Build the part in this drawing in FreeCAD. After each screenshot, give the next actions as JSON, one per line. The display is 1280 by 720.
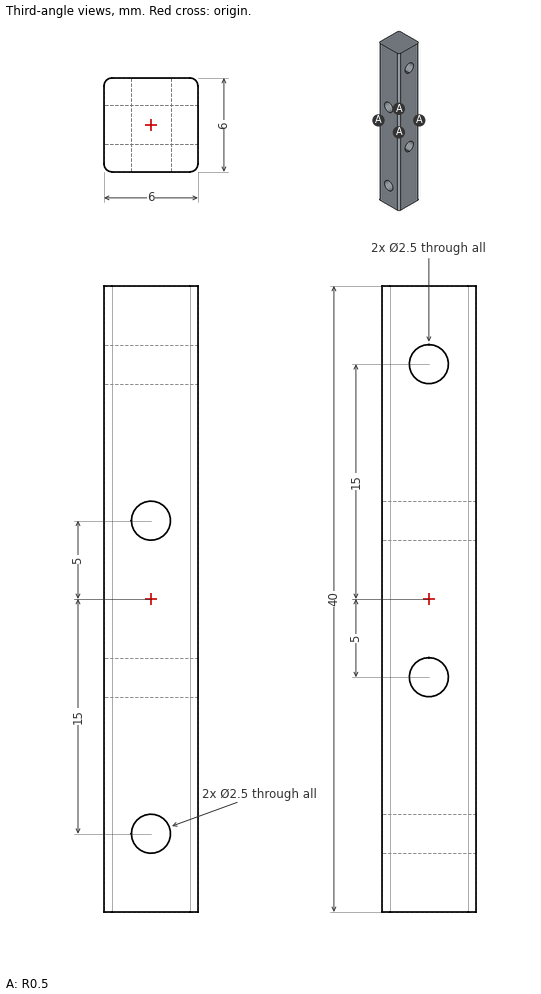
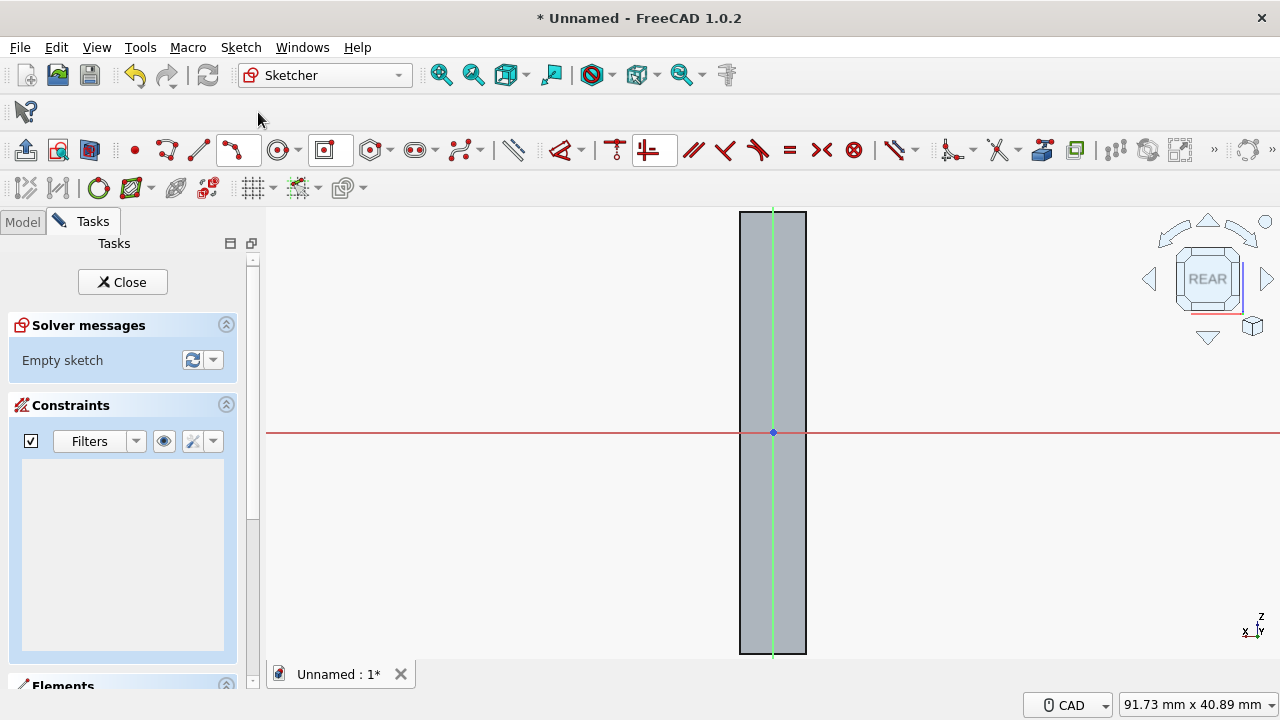
{"action": "scroll", "coordinate": [395, 235], "scroll_direction": "down", "scroll_amount": 1}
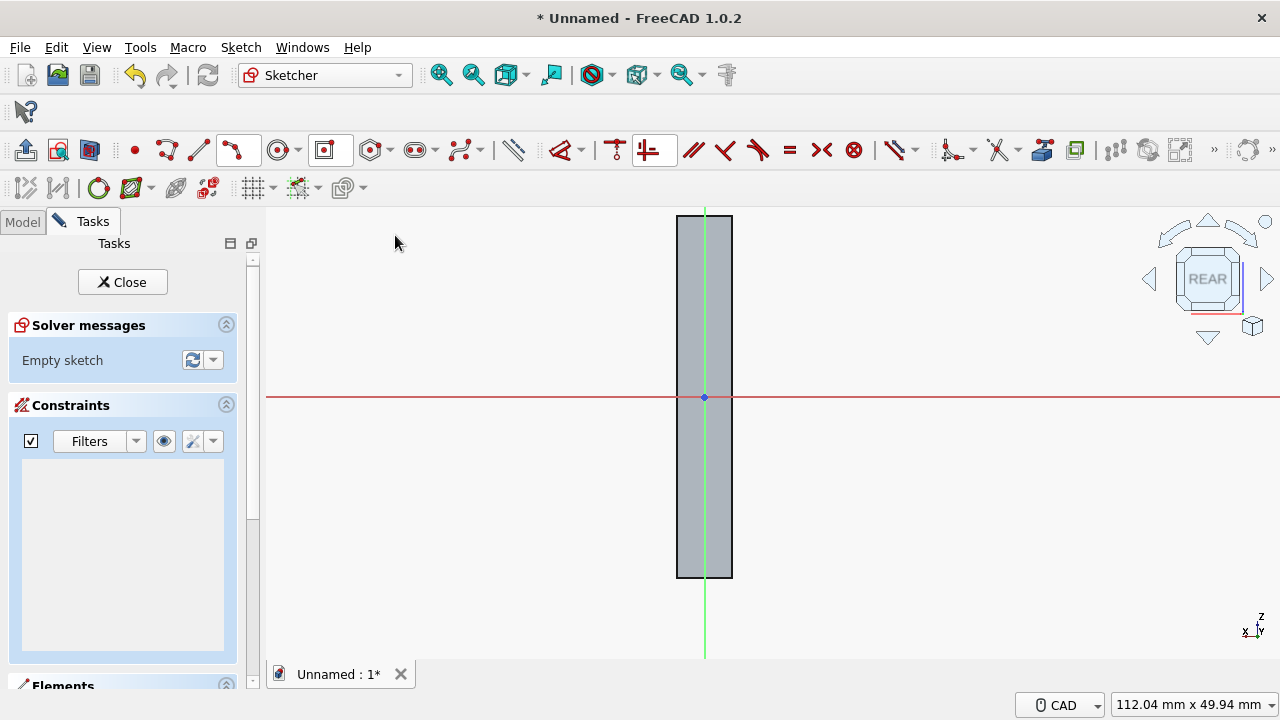
{"action": "scroll", "coordinate": [705, 461], "scroll_direction": "up", "scroll_amount": 2}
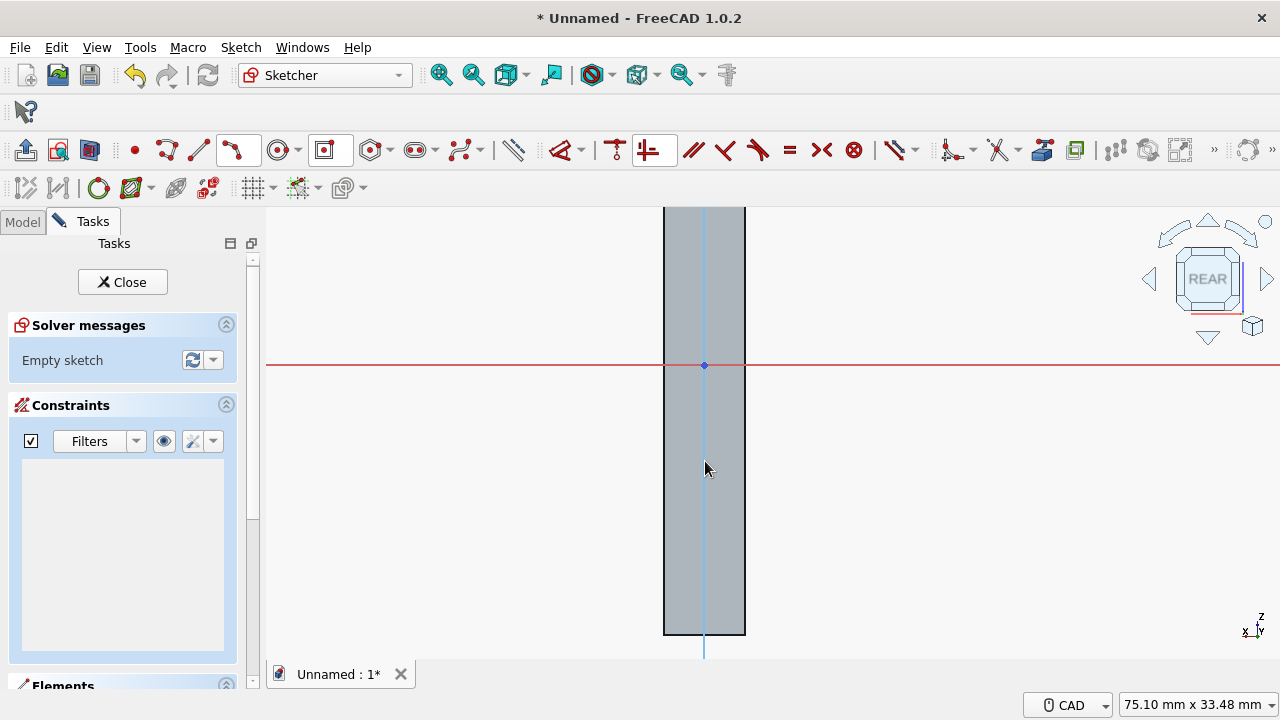
{"action": "left_click", "coordinate": [278, 150]}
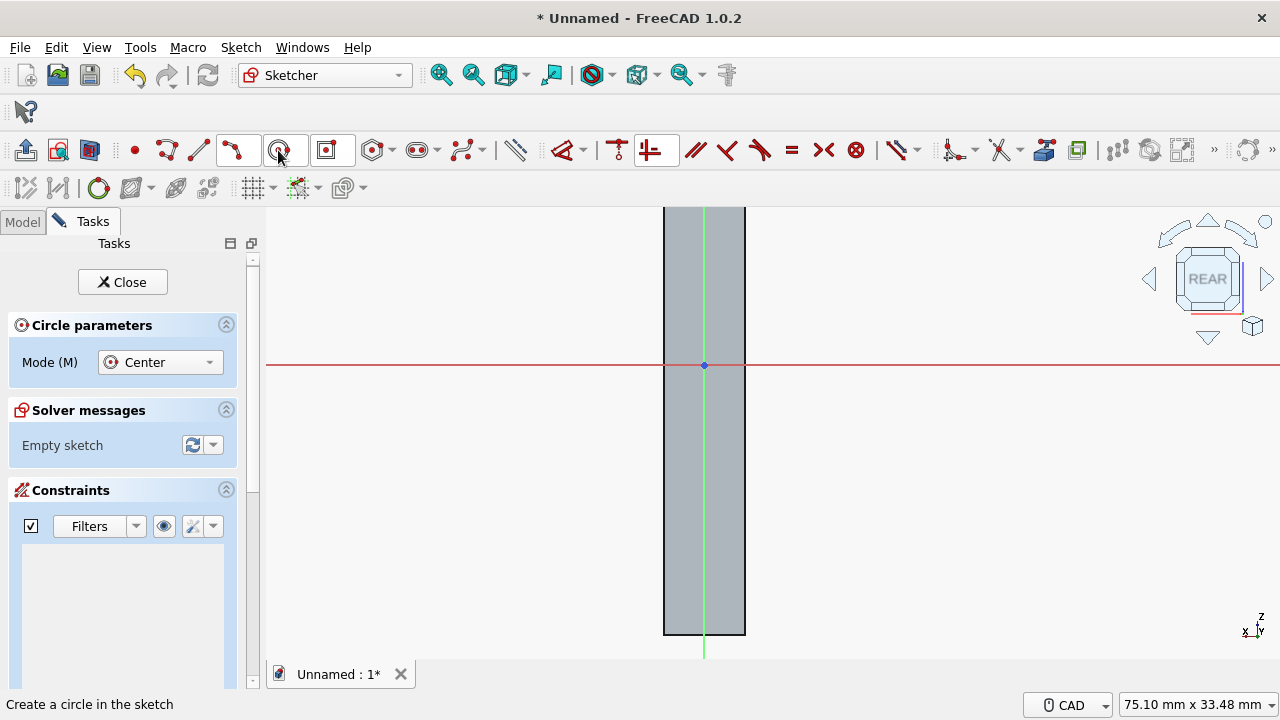
{"action": "scroll", "coordinate": [704, 568], "scroll_direction": "up", "scroll_amount": 2}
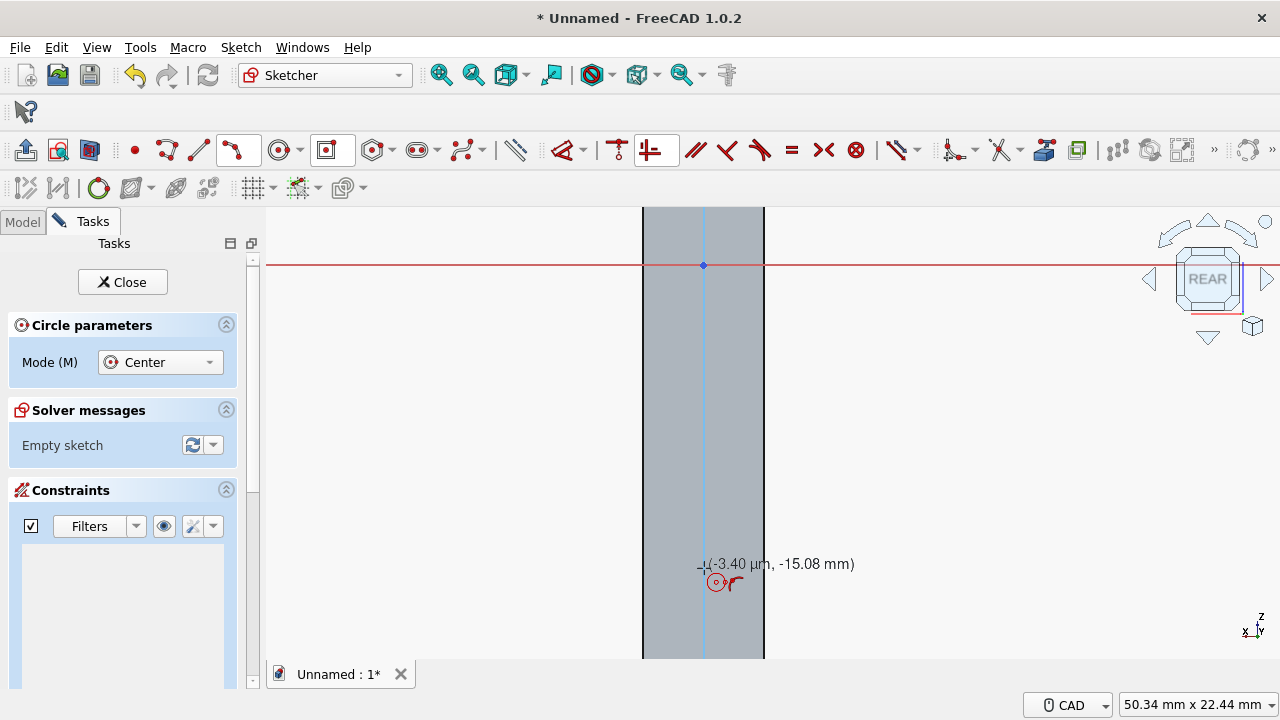
{"action": "left_click", "coordinate": [704, 568]}
{"action": "left_click", "coordinate": [722, 550]}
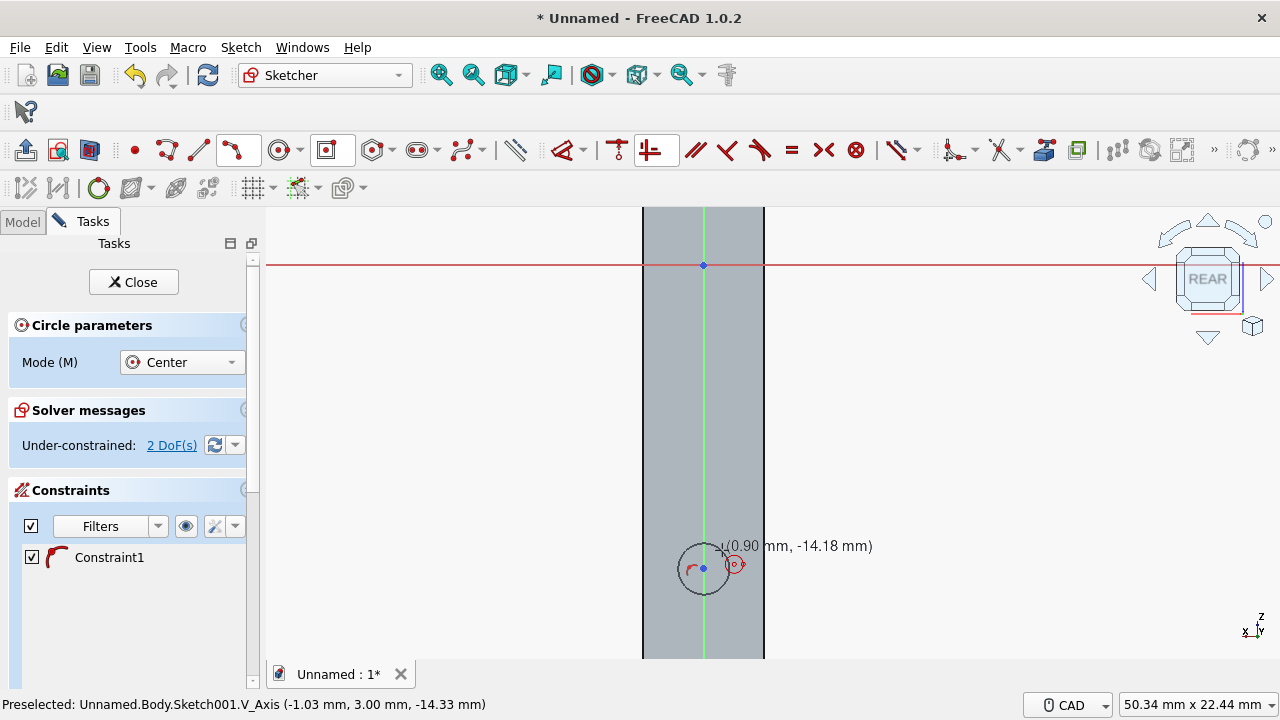
{"action": "scroll", "coordinate": [706, 569], "scroll_direction": "down", "scroll_amount": 2}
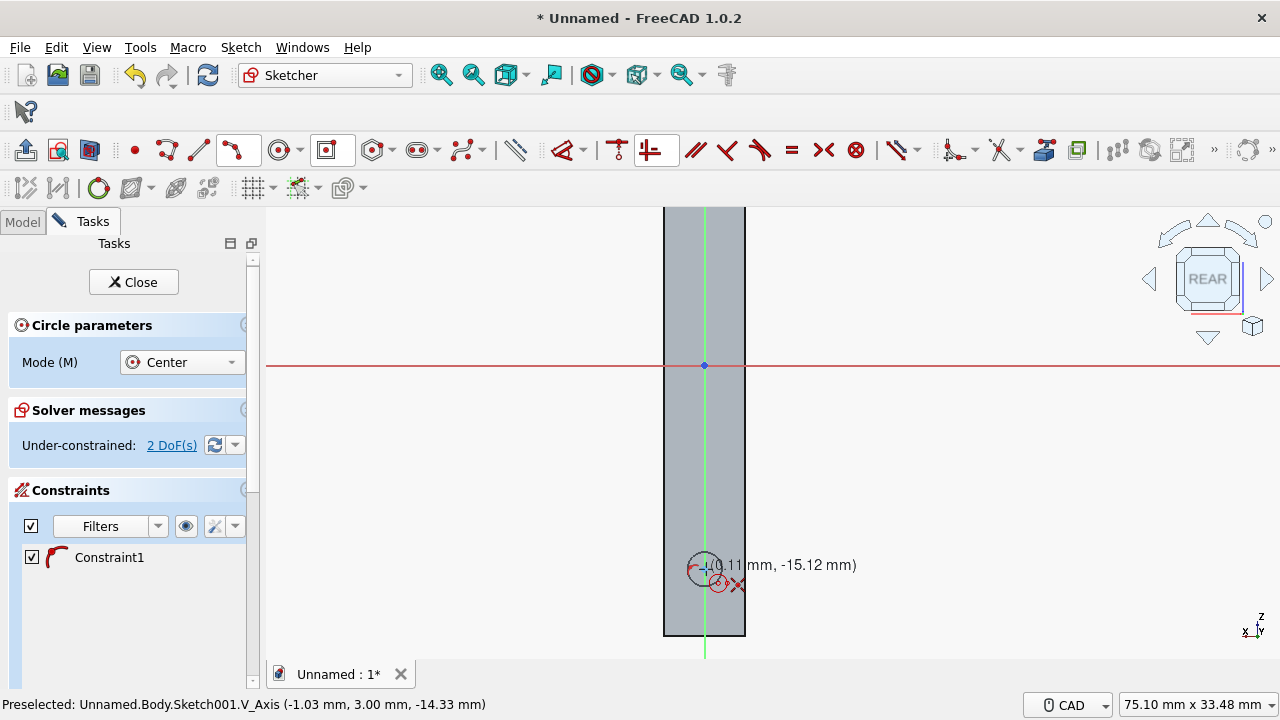
{"action": "scroll", "coordinate": [705, 298], "scroll_direction": "up", "scroll_amount": 2}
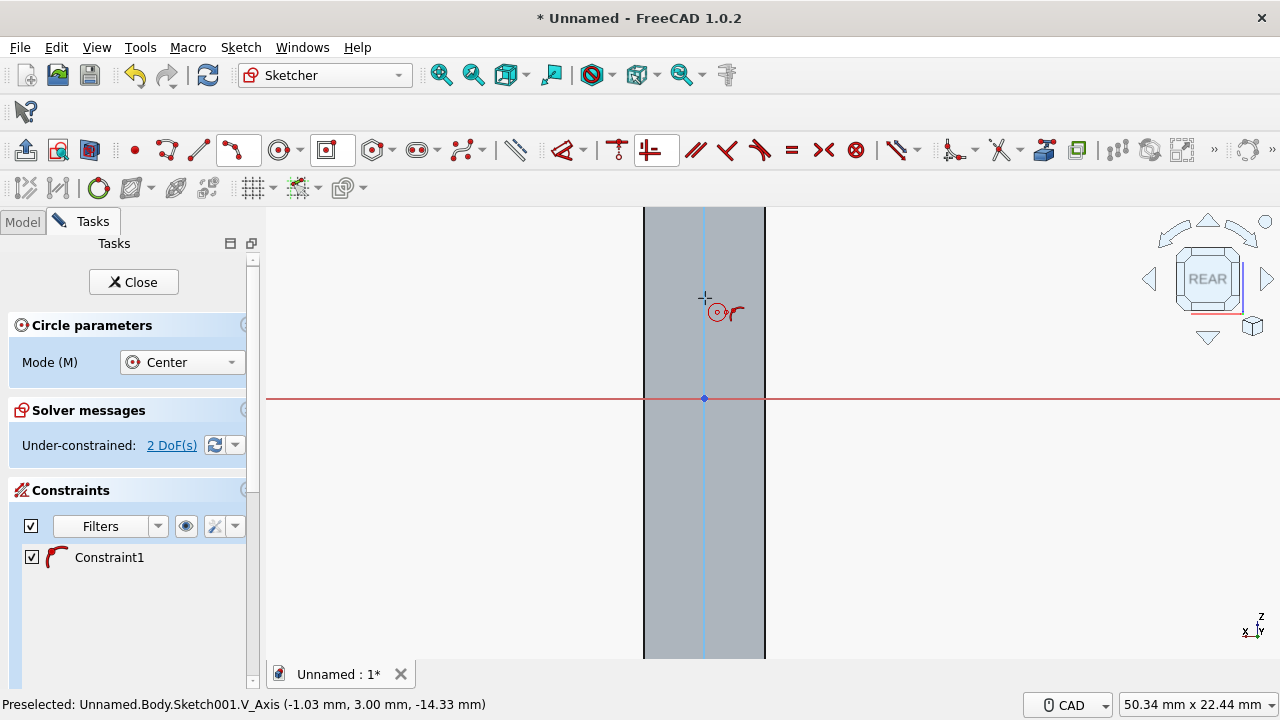
{"action": "left_click", "coordinate": [704, 298]}
{"action": "left_click", "coordinate": [722, 280]}
{"action": "key", "text": "Escape"}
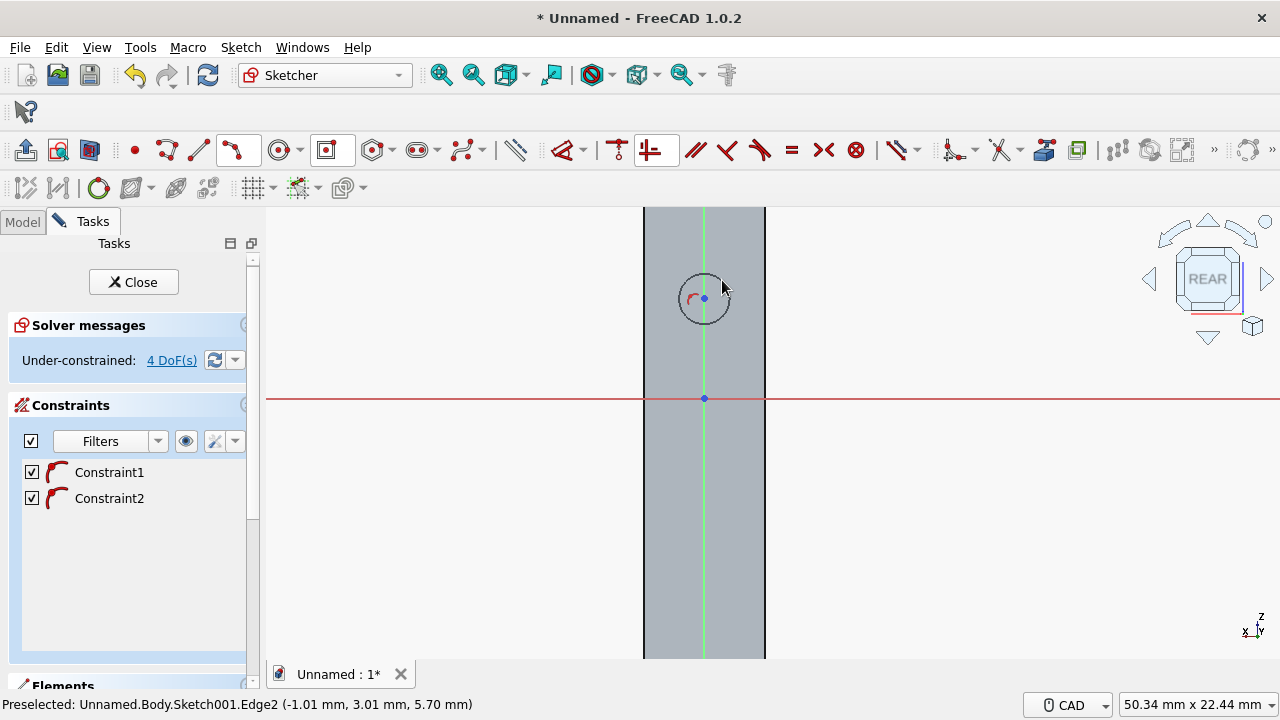
{"action": "scroll", "coordinate": [705, 297], "scroll_direction": "down", "scroll_amount": 2}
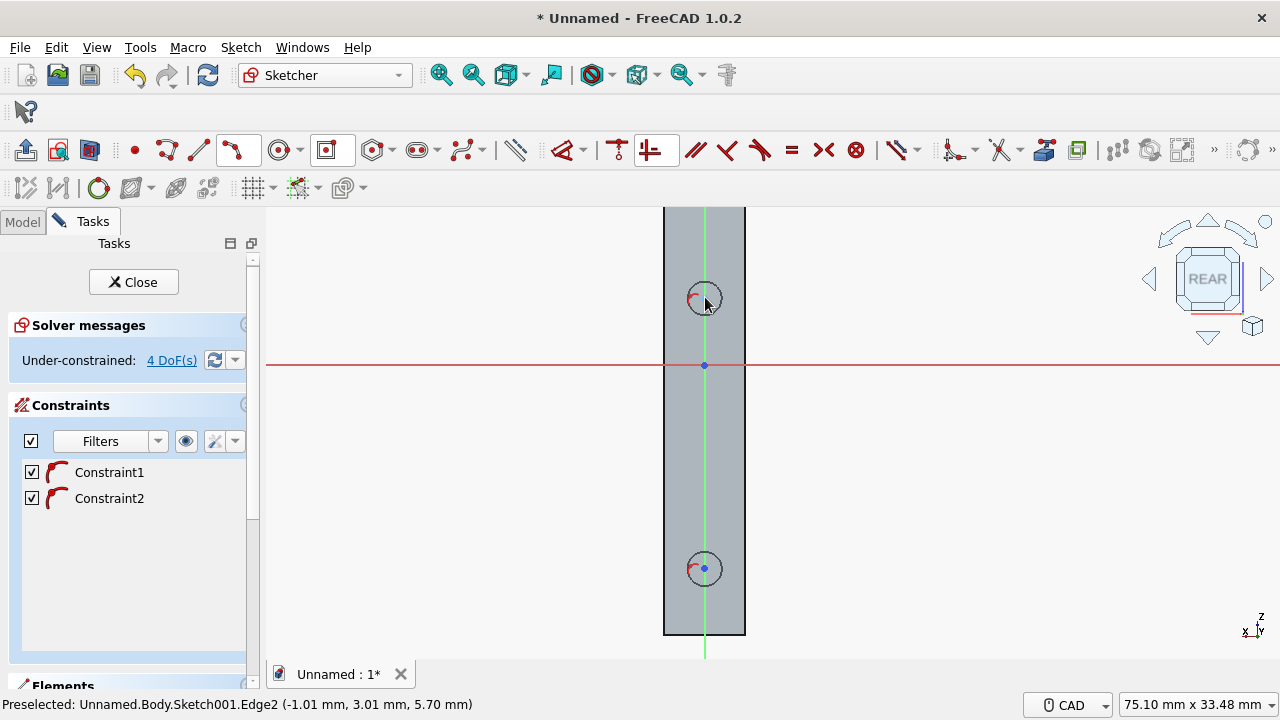
{"action": "left_click", "coordinate": [717, 557]}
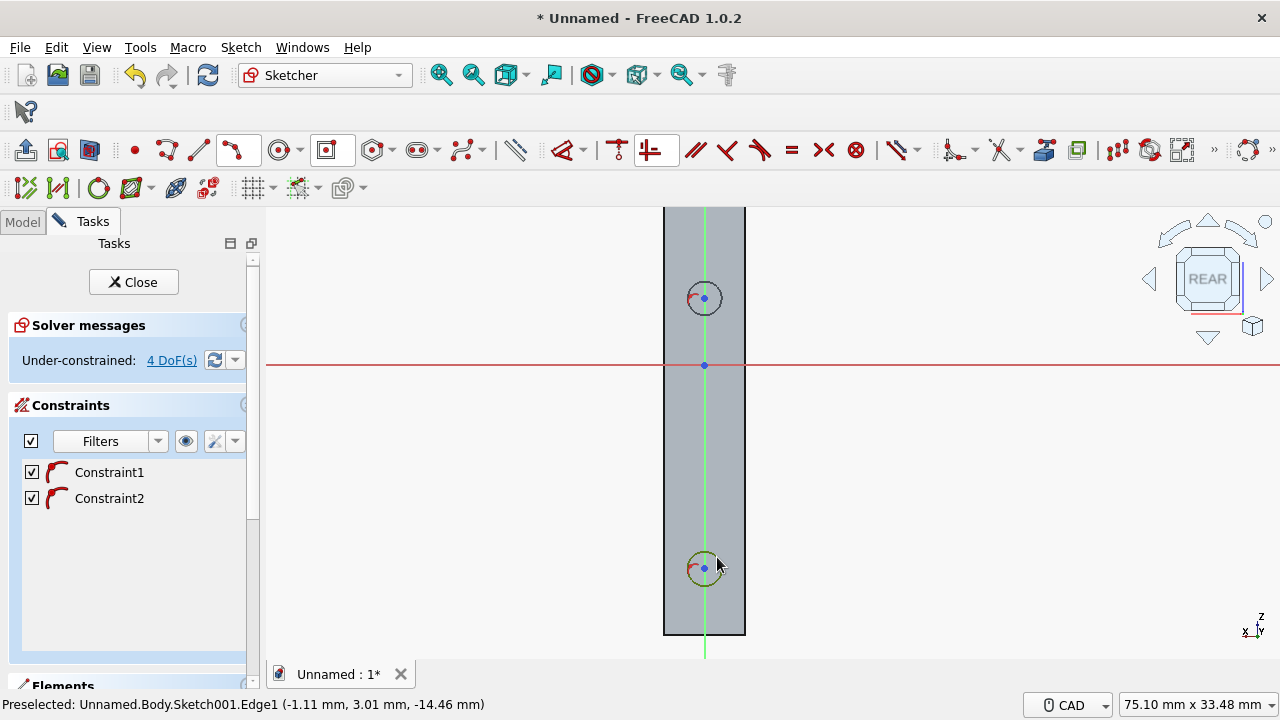
{"action": "left_click", "coordinate": [717, 286]}